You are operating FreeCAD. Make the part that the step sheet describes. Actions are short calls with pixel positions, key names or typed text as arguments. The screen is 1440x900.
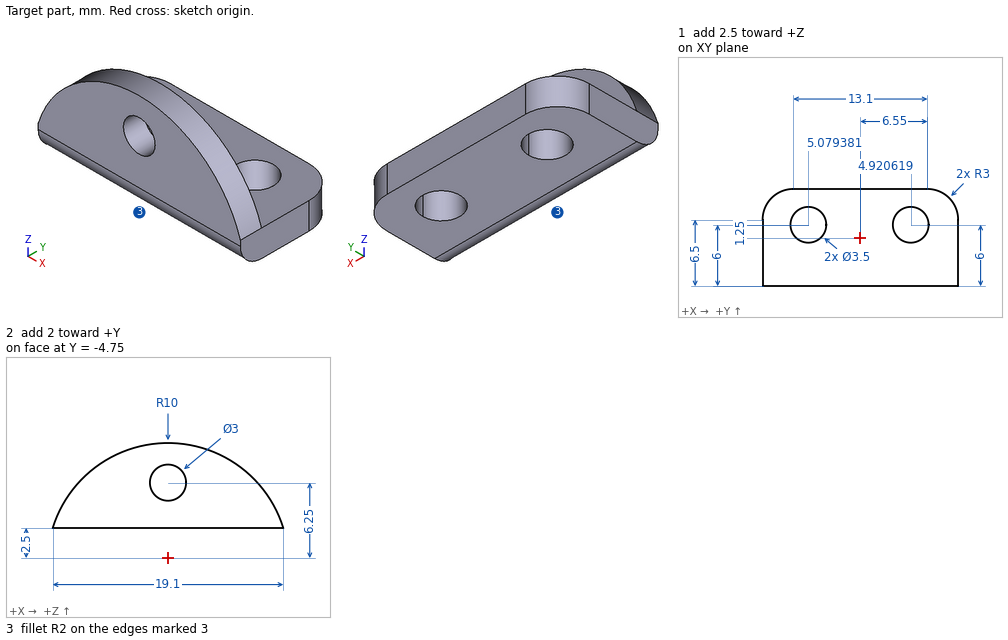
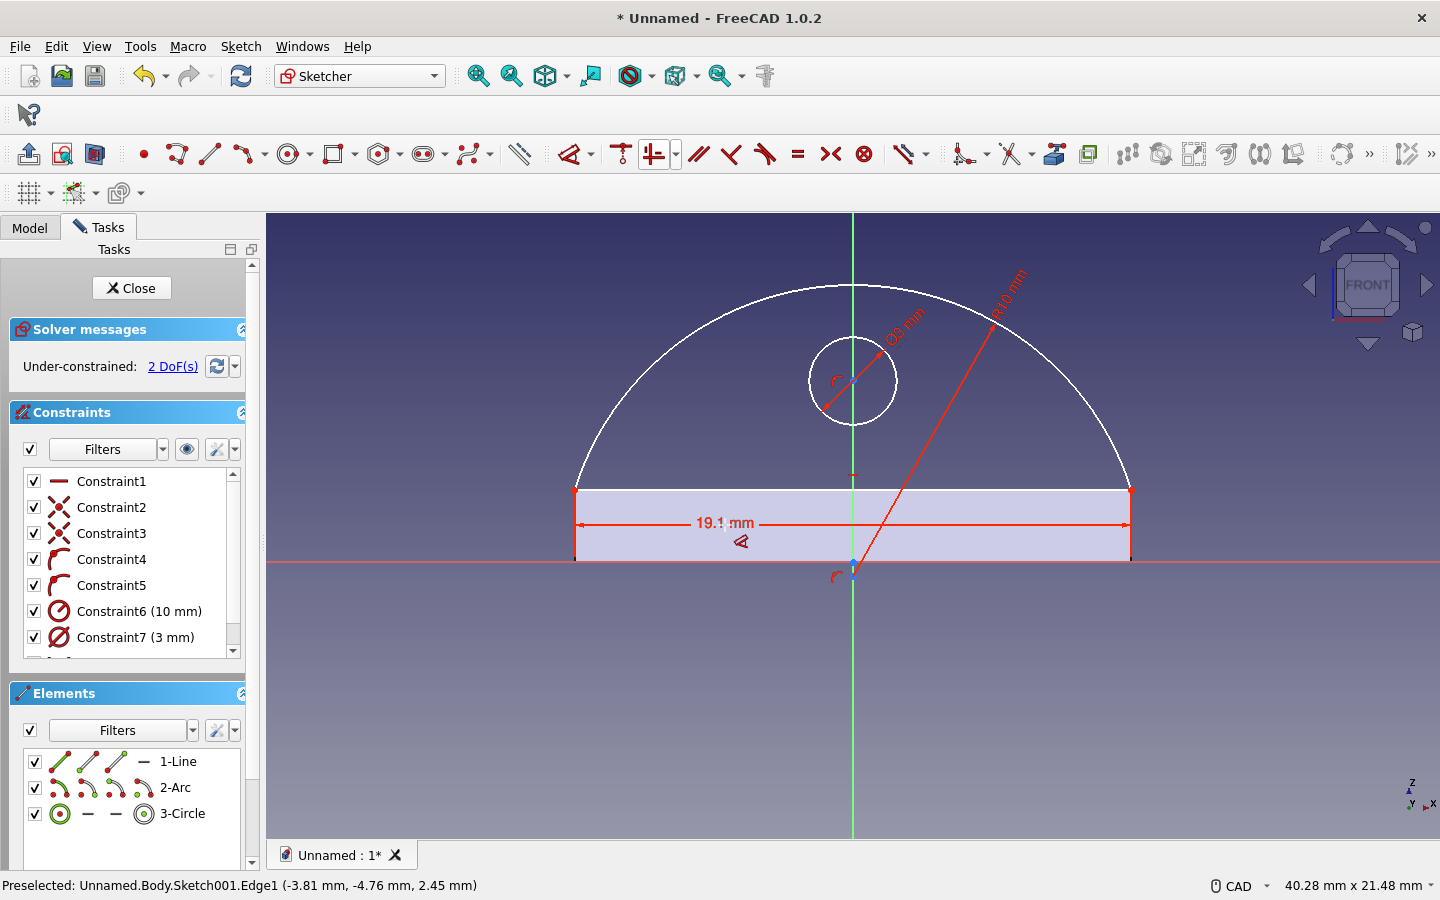
click(575, 490)
click(541, 526)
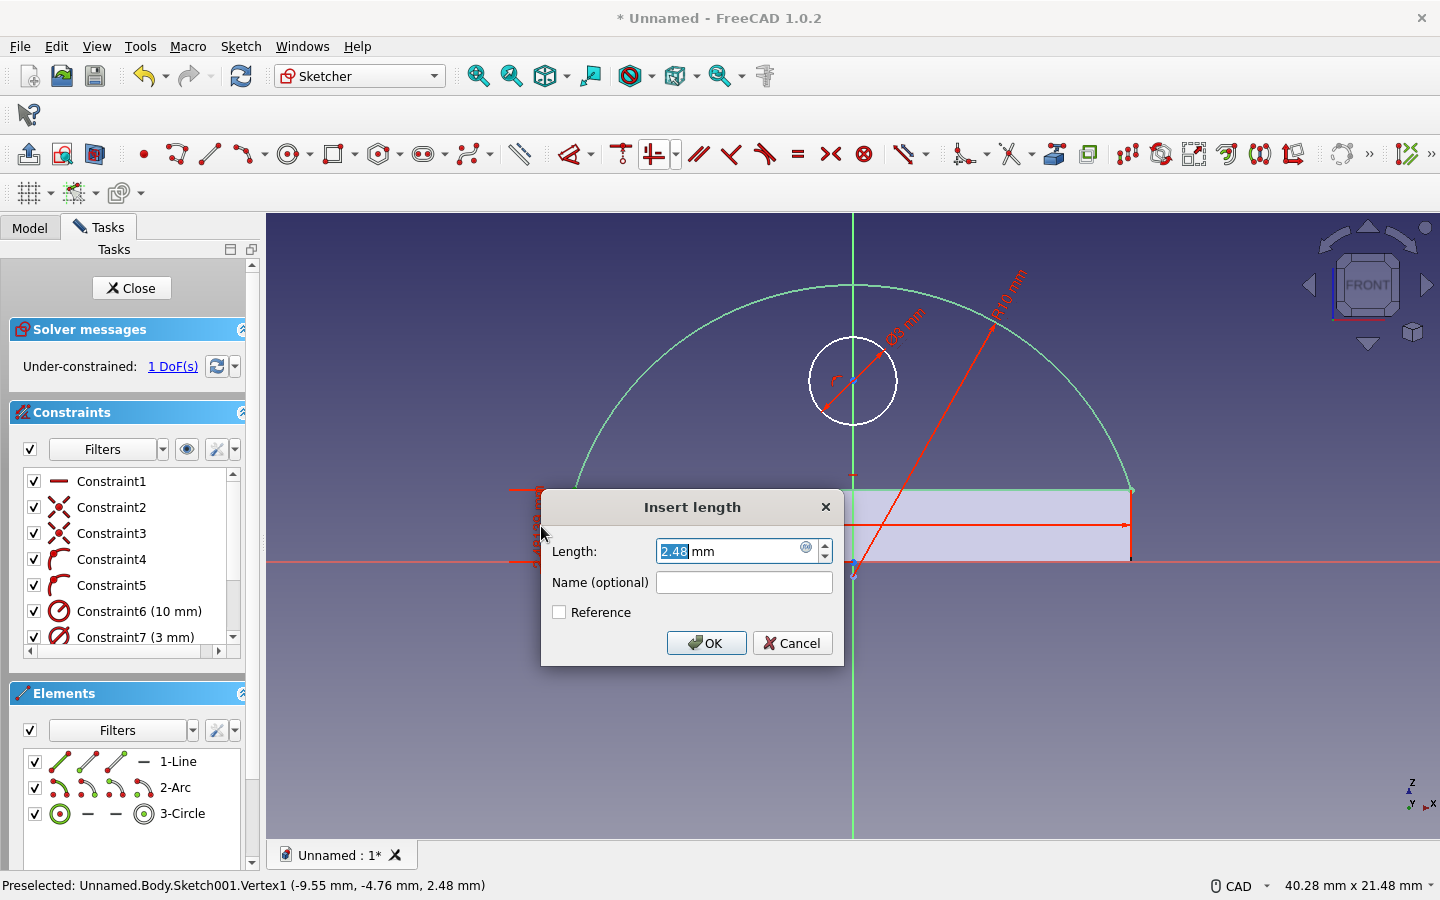
text(2.5)
key(Return)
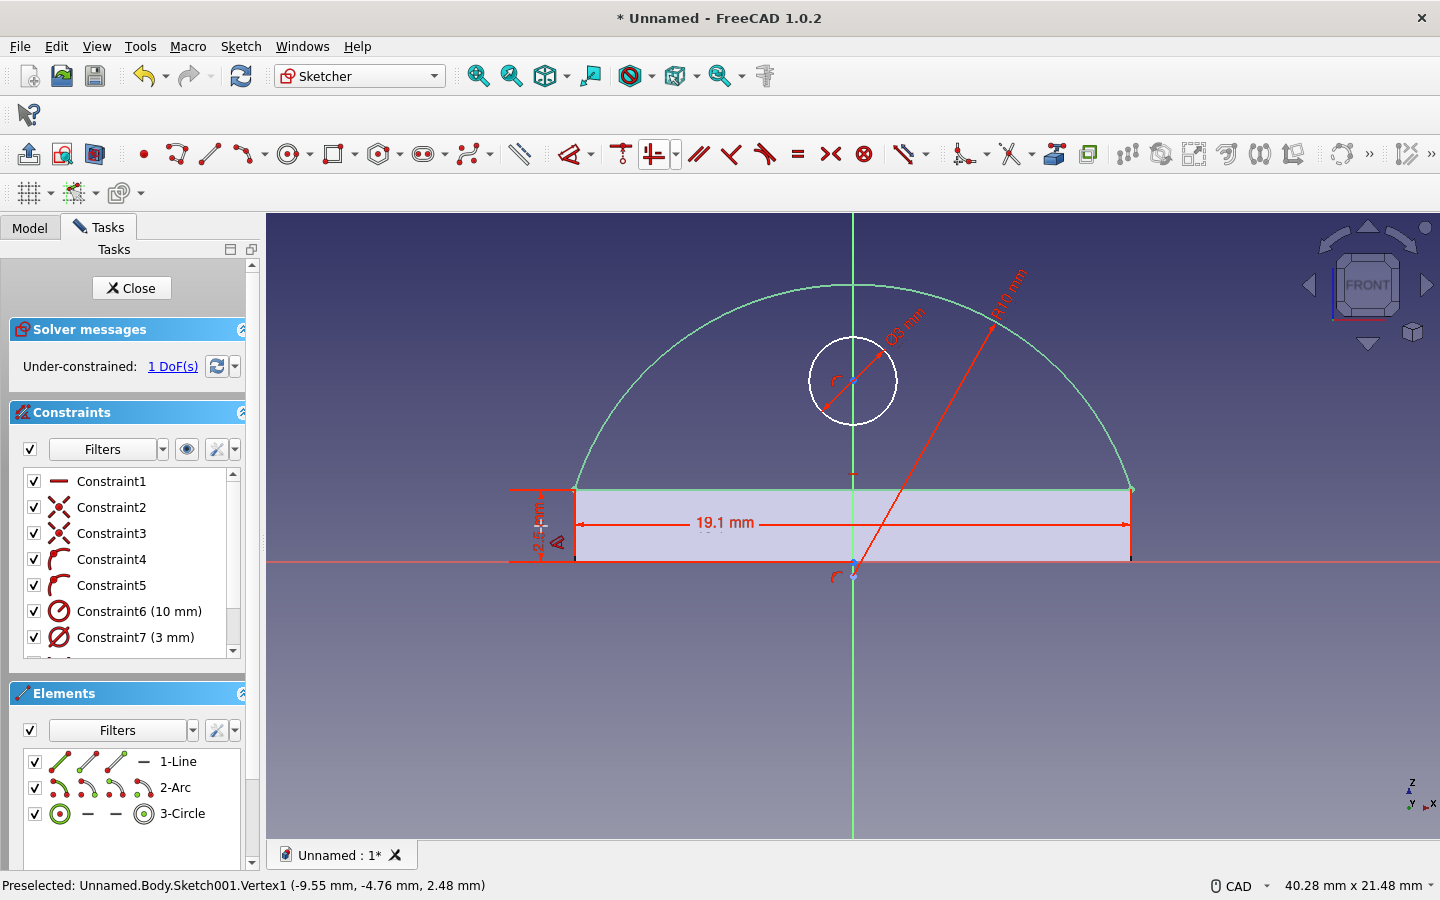
click(853, 381)
click(887, 472)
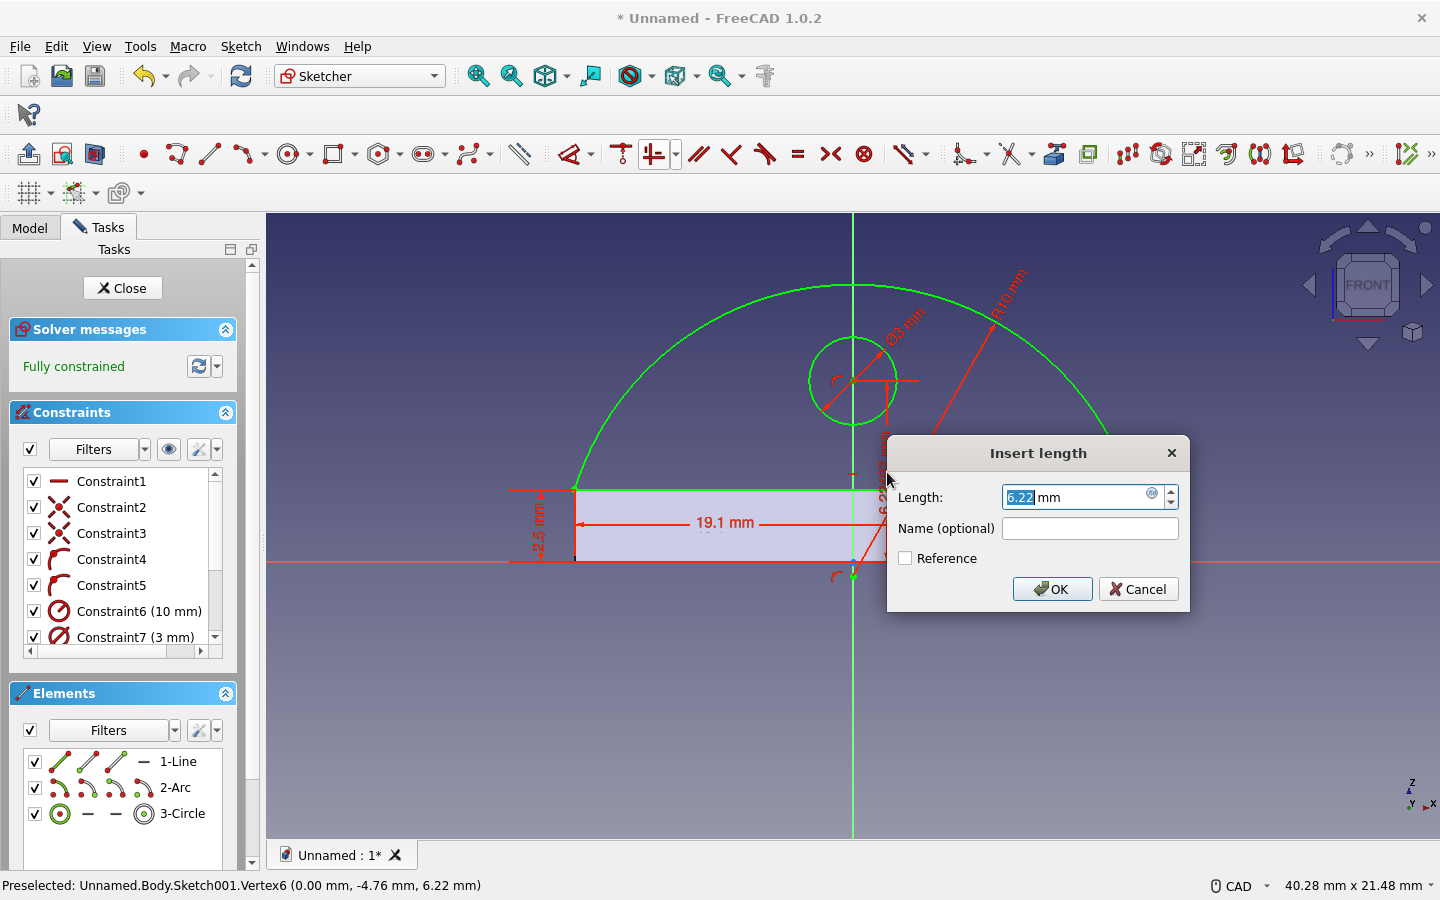
text(6.25)
key(Return)
key(Escape)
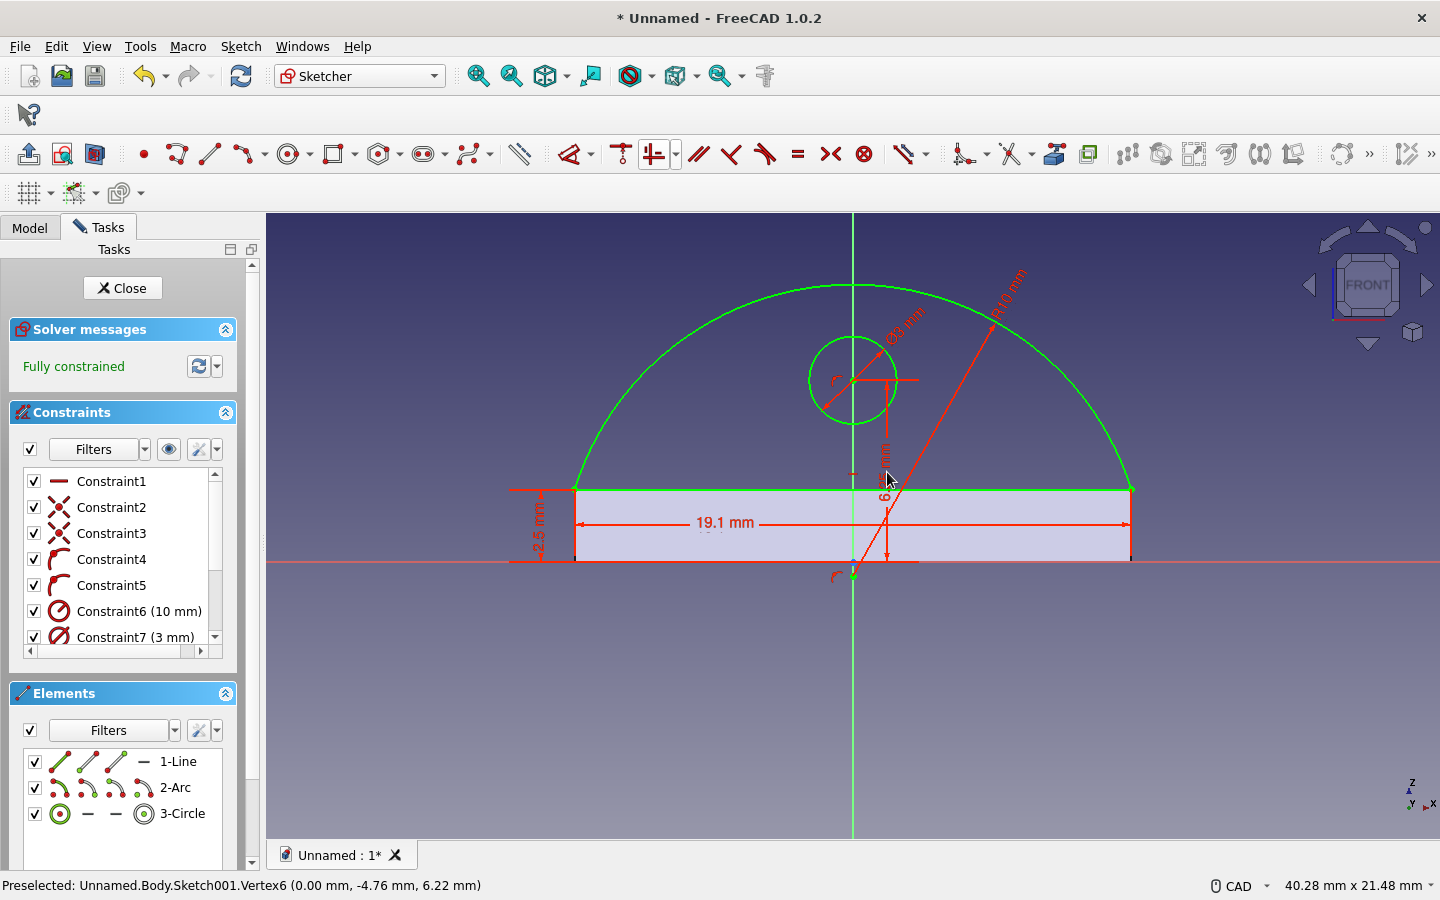
click(123, 288)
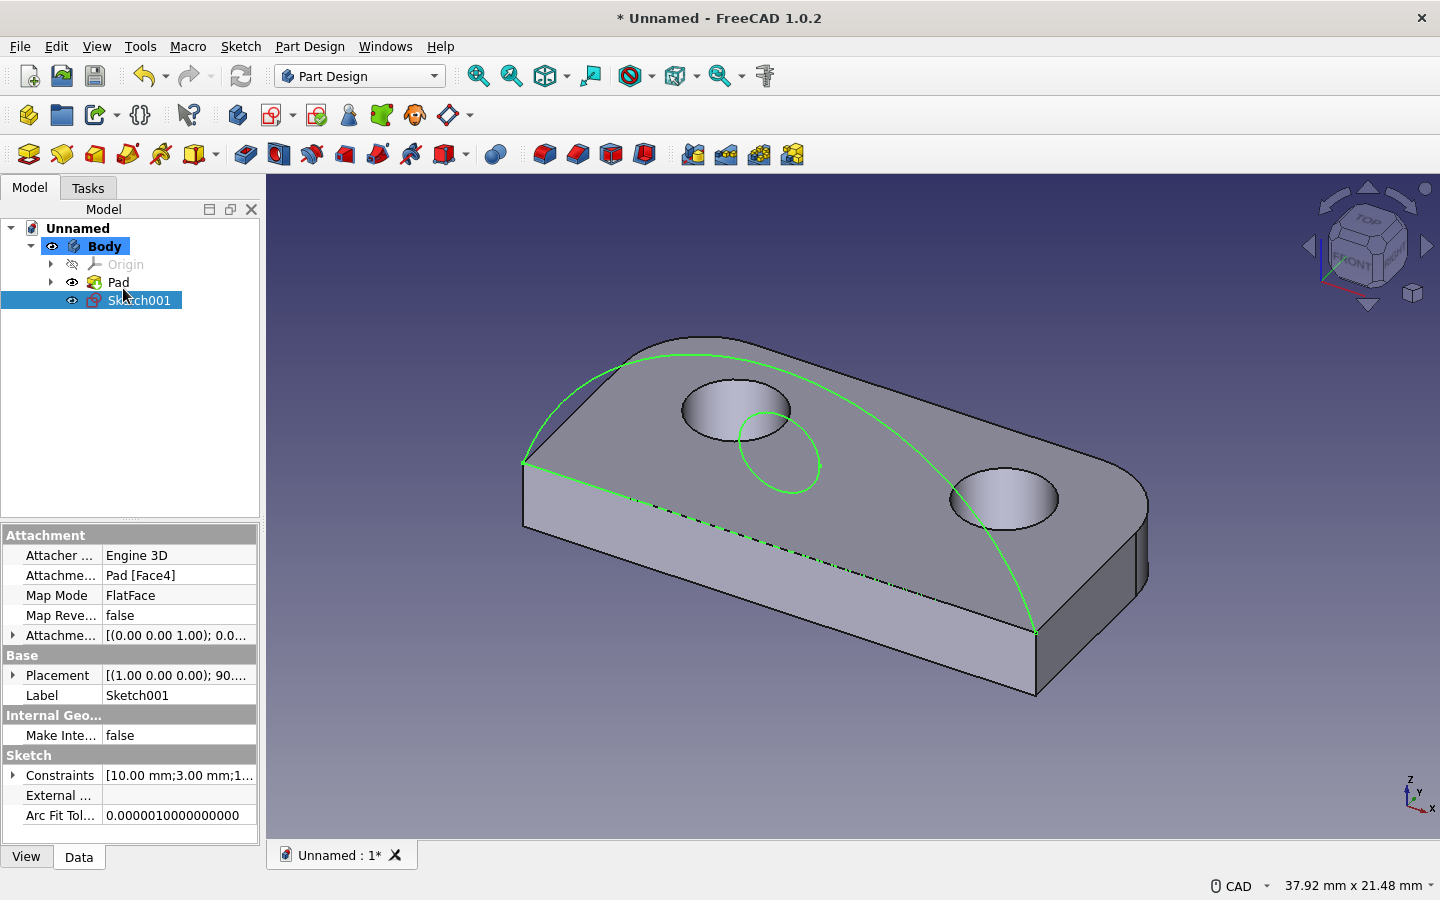
click(29, 154)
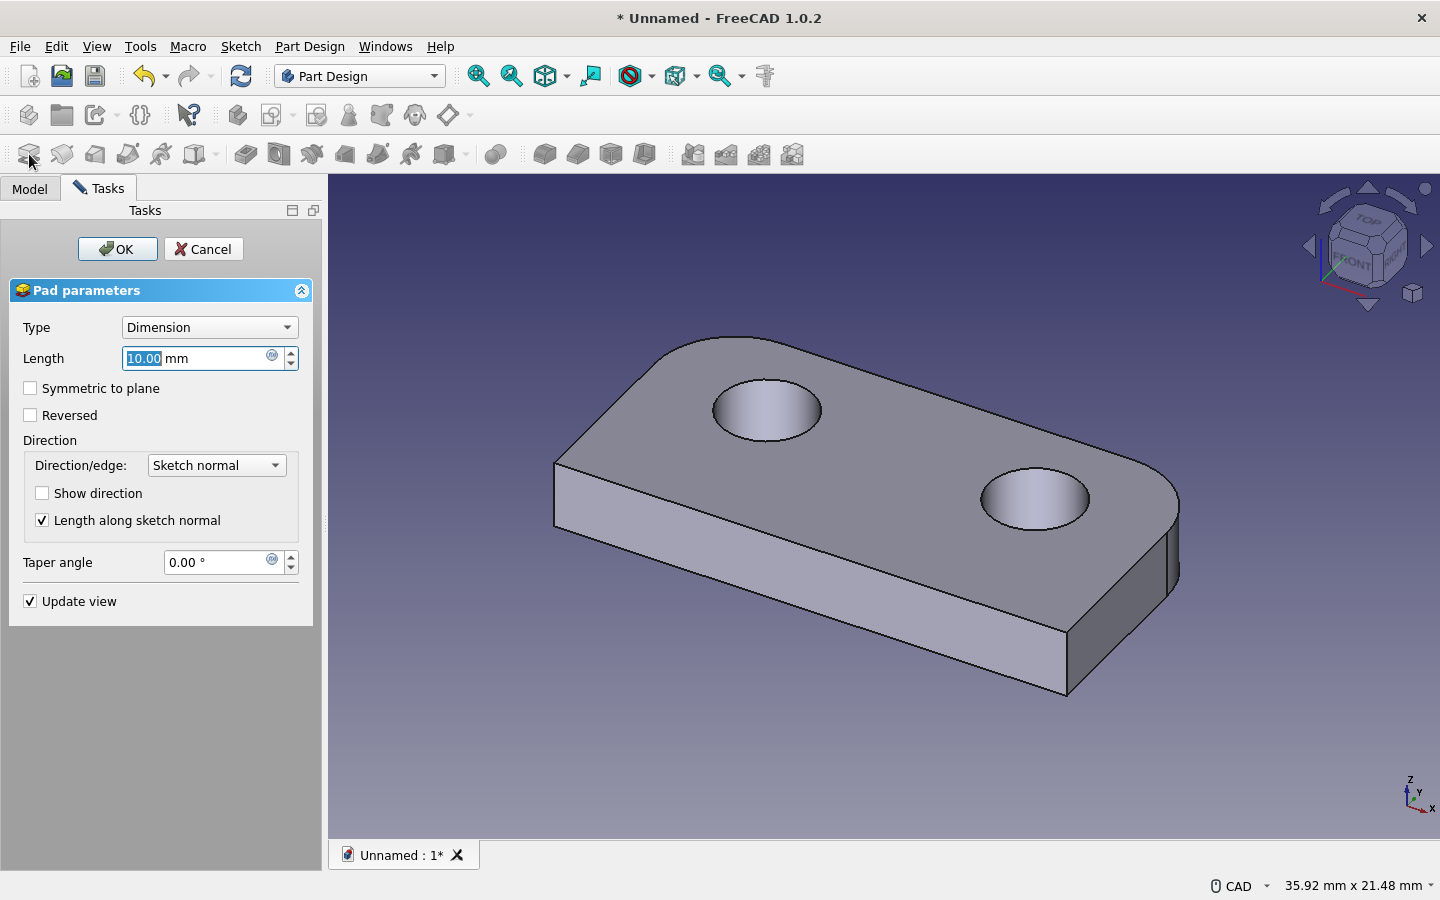
text(2)
key(Tab)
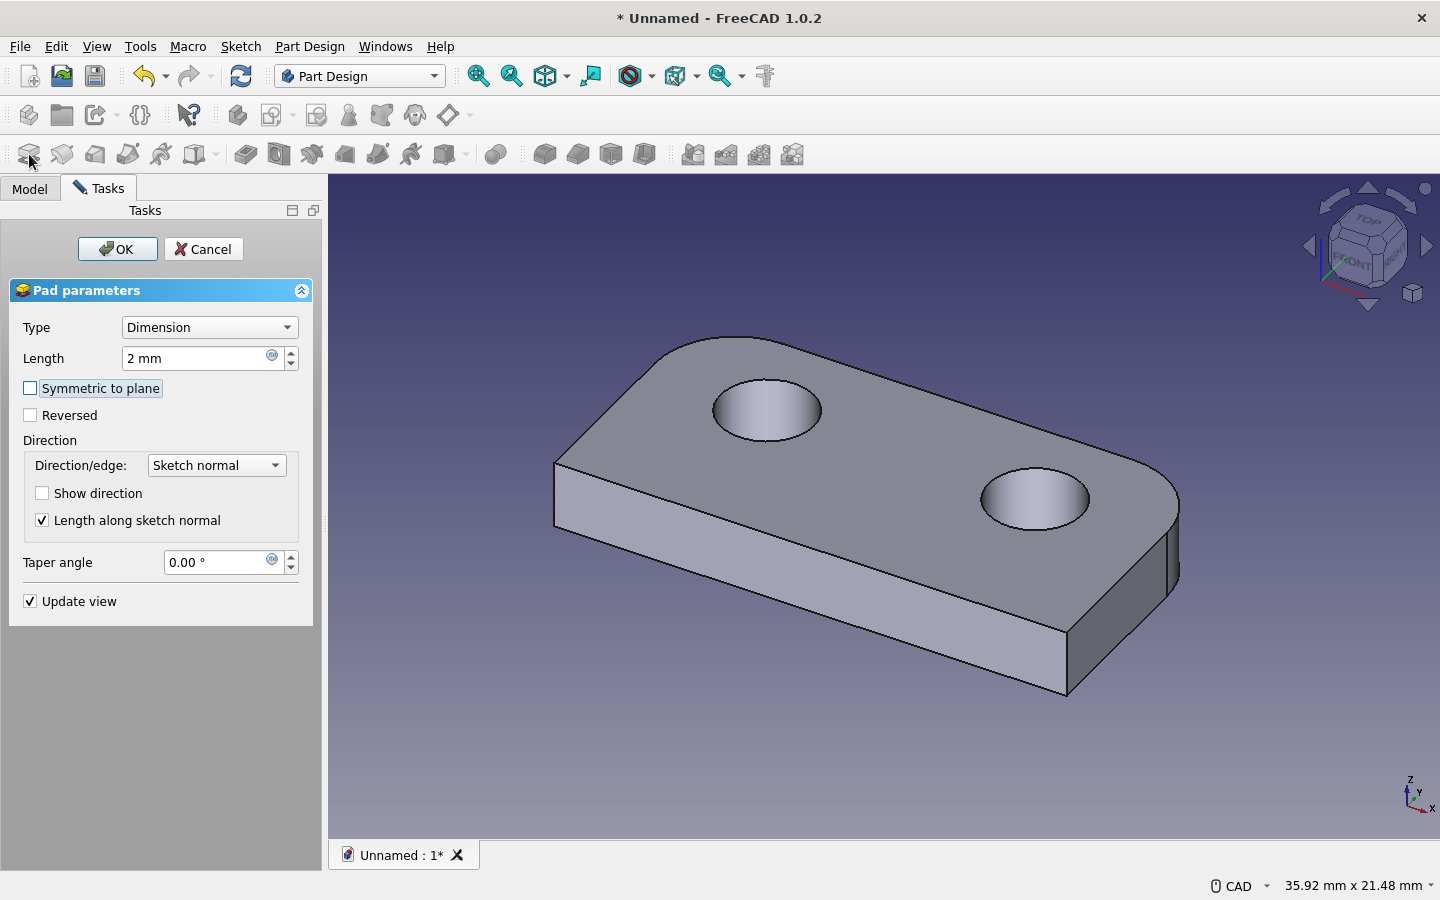
click(31, 415)